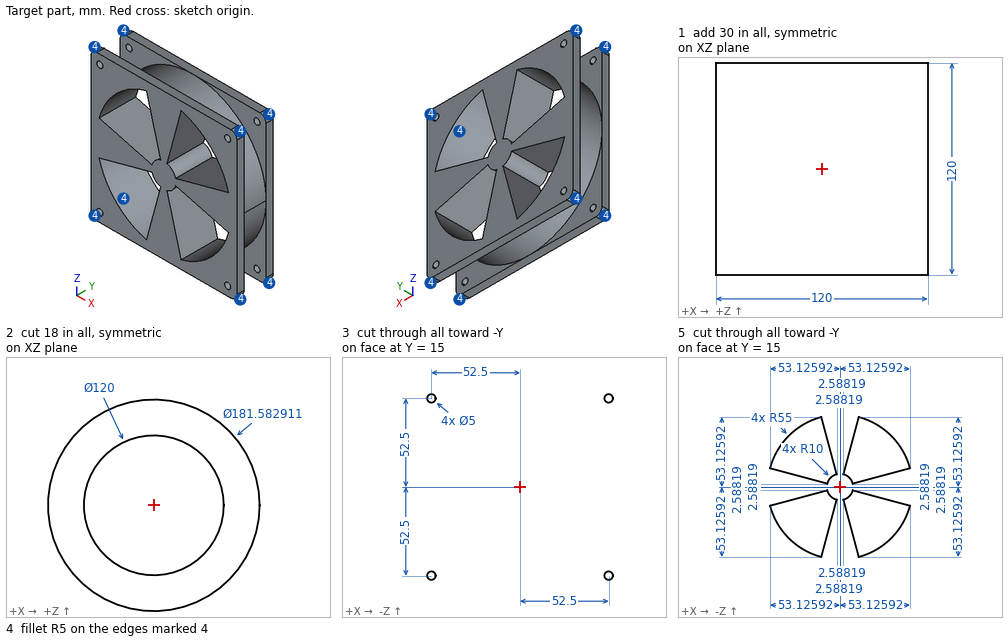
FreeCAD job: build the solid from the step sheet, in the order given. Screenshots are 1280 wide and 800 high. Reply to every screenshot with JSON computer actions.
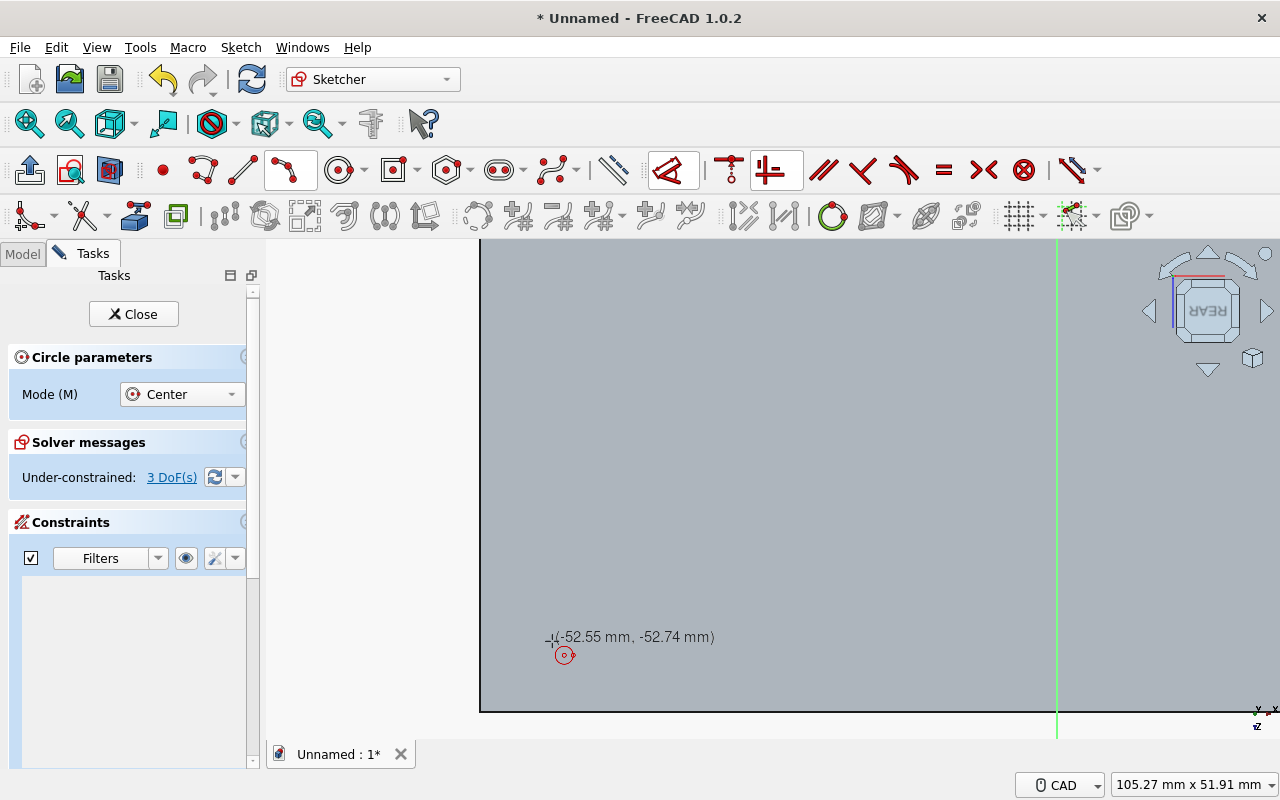
{"action": "left_click", "coordinate": [552, 640]}
{"action": "left_click", "coordinate": [569, 623]}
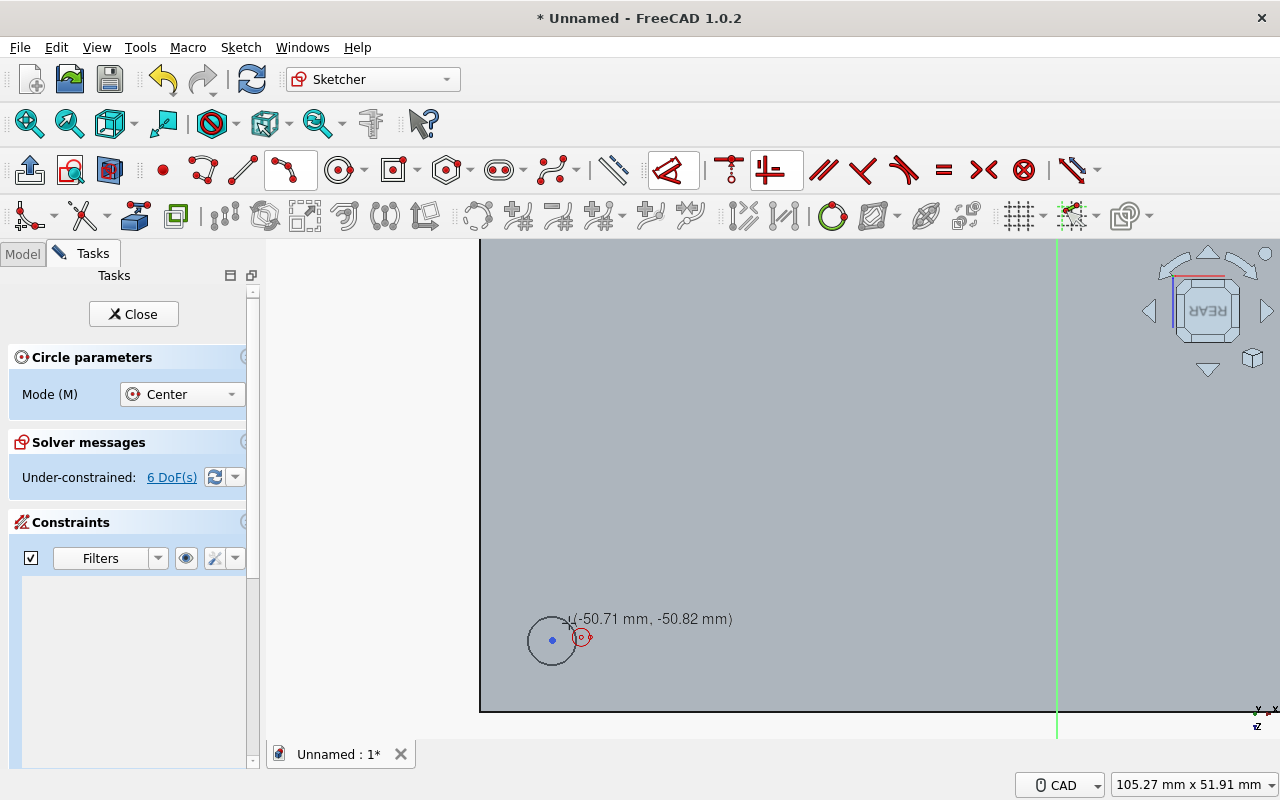
{"action": "scroll", "coordinate": [552, 642], "scroll_direction": "down", "scroll_amount": 6}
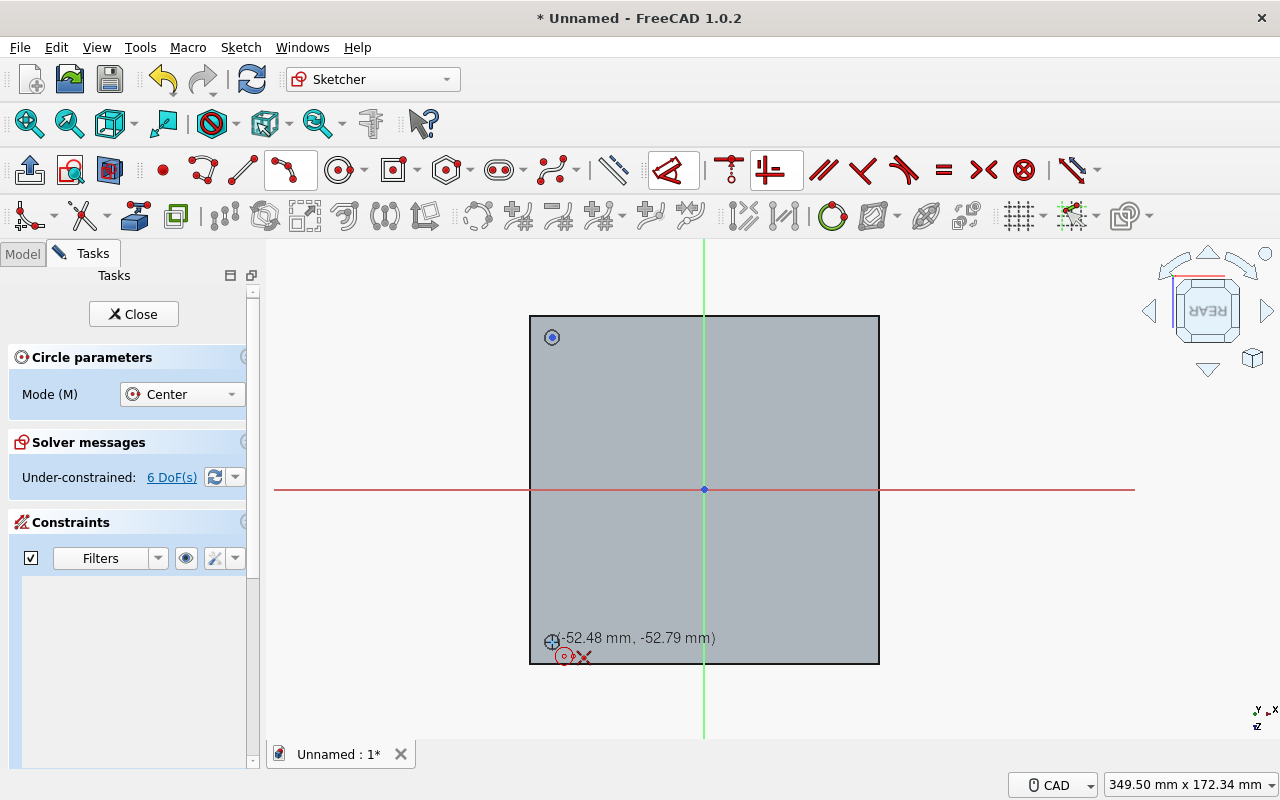
{"action": "scroll", "coordinate": [857, 642], "scroll_direction": "up", "scroll_amount": 6}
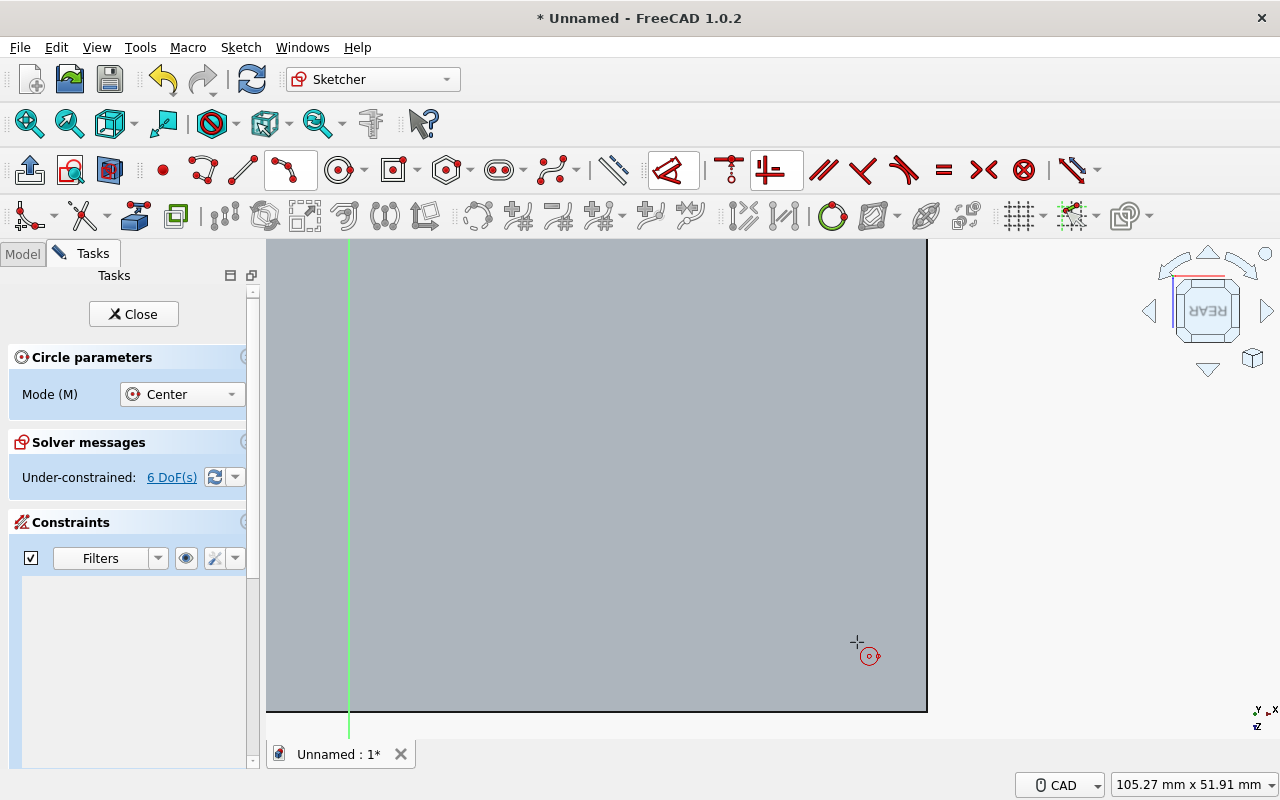
{"action": "left_click", "coordinate": [855, 640]}
{"action": "left_click", "coordinate": [872, 623]}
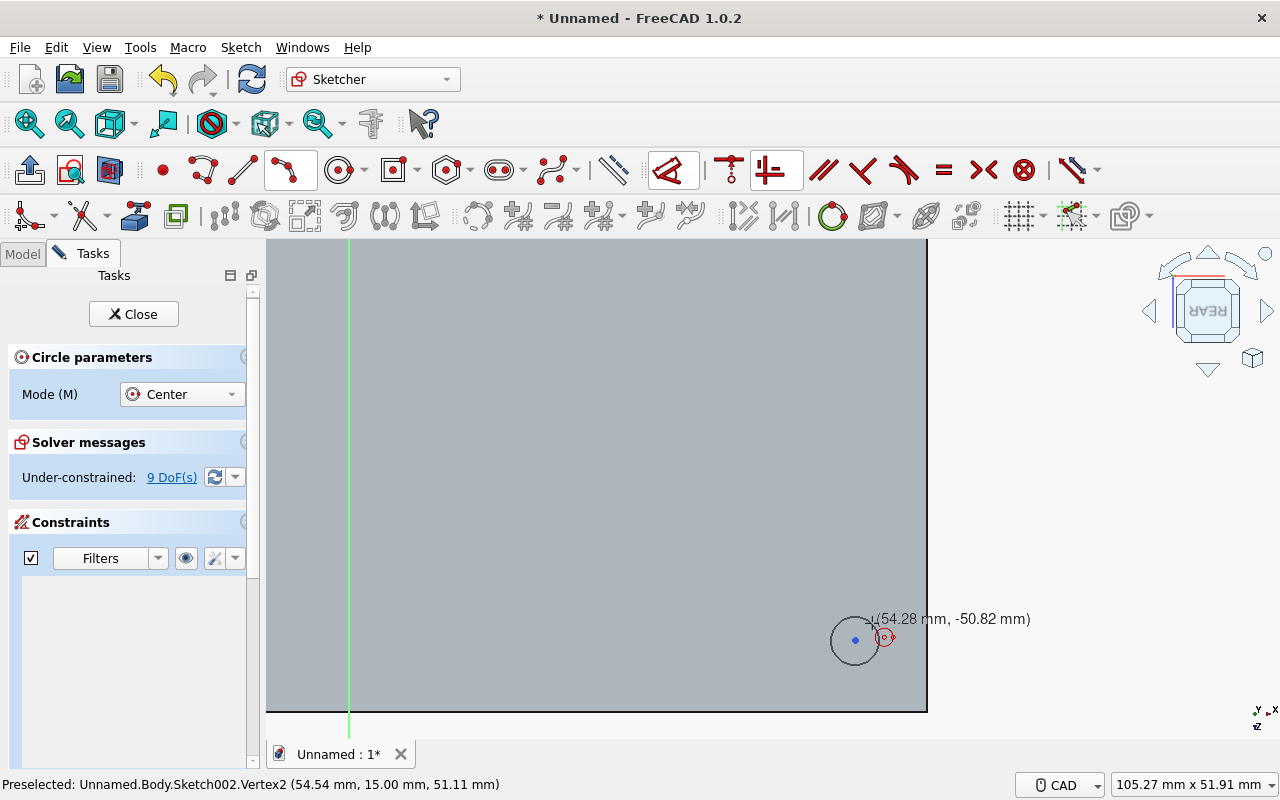
{"action": "scroll", "coordinate": [858, 642], "scroll_direction": "down", "scroll_amount": 6}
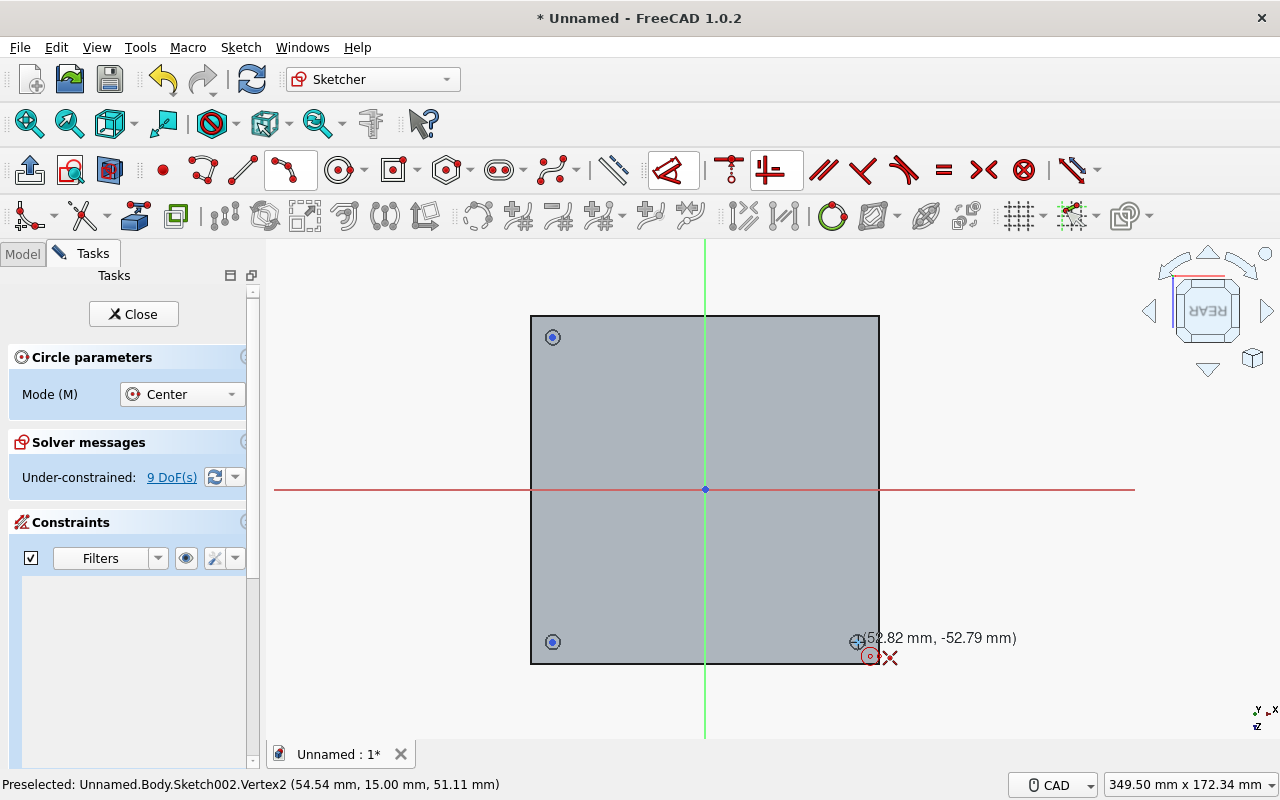
{"action": "scroll", "coordinate": [857, 337], "scroll_direction": "up", "scroll_amount": 6}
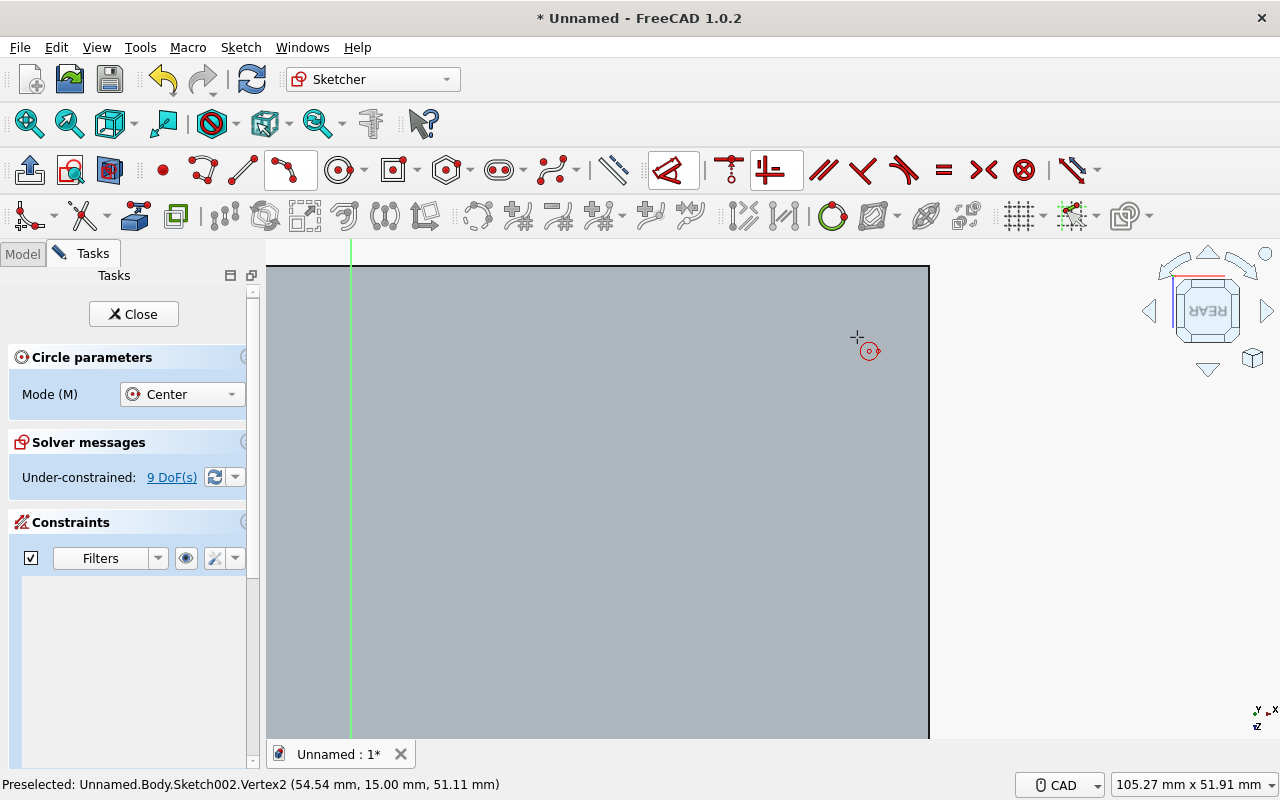
{"action": "left_click", "coordinate": [857, 338]}
{"action": "left_click", "coordinate": [874, 321]}
{"action": "key", "text": "Escape"}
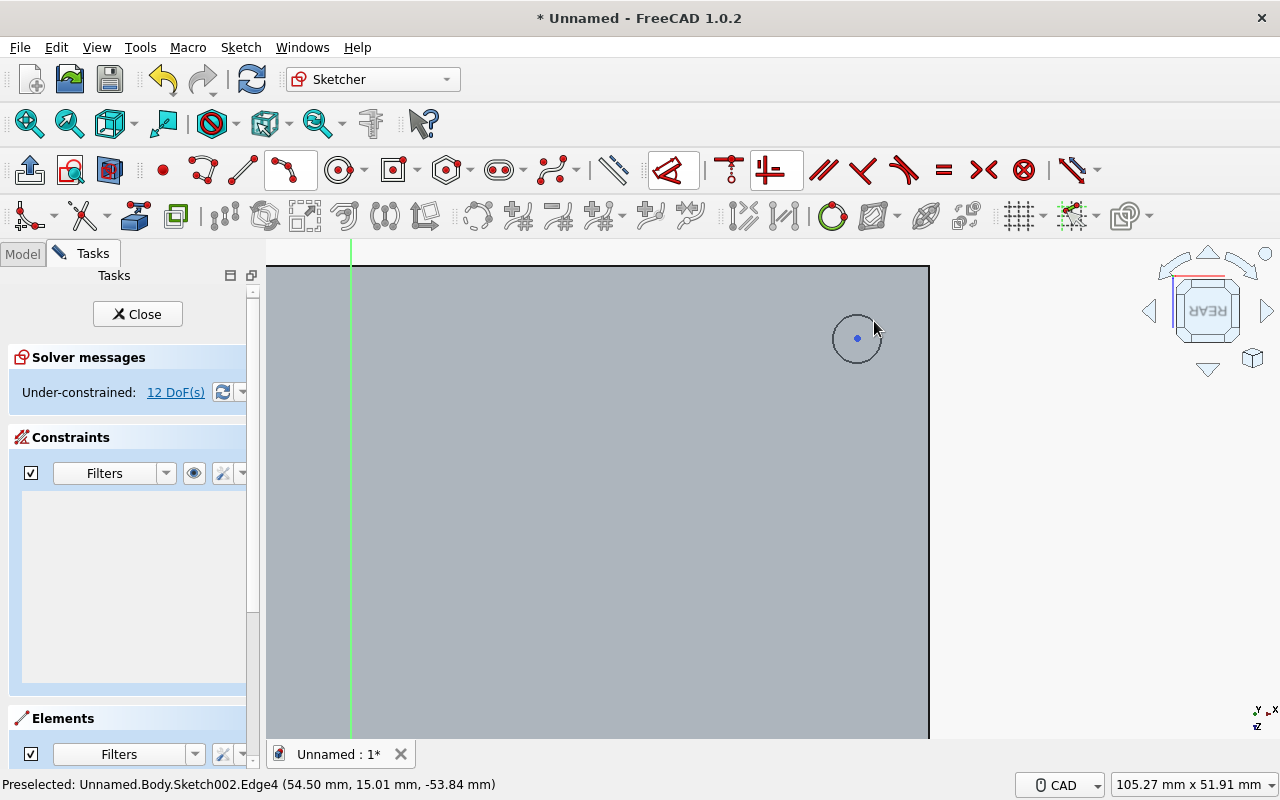
{"action": "scroll", "coordinate": [857, 336], "scroll_direction": "down", "scroll_amount": 6}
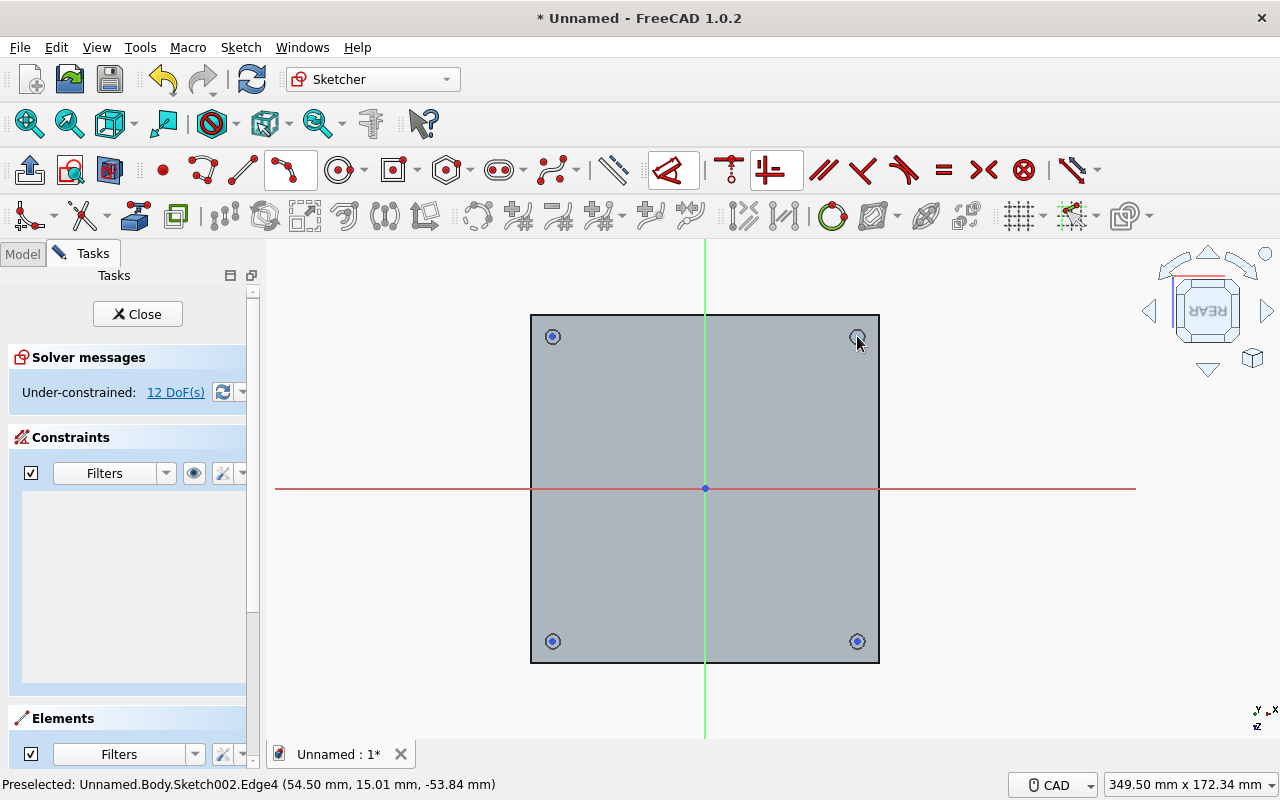
{"action": "scroll", "coordinate": [558, 332], "scroll_direction": "up", "scroll_amount": 4}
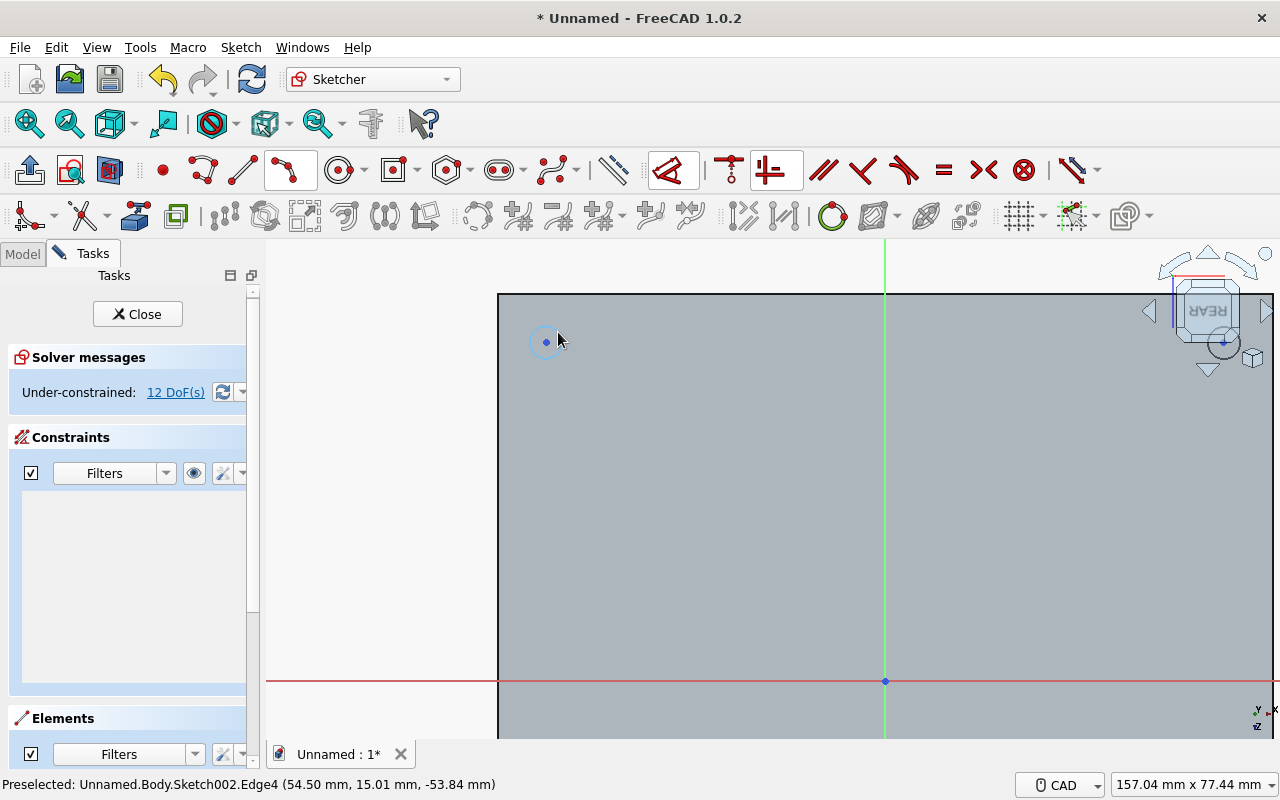
{"action": "left_click", "coordinate": [557, 331]}